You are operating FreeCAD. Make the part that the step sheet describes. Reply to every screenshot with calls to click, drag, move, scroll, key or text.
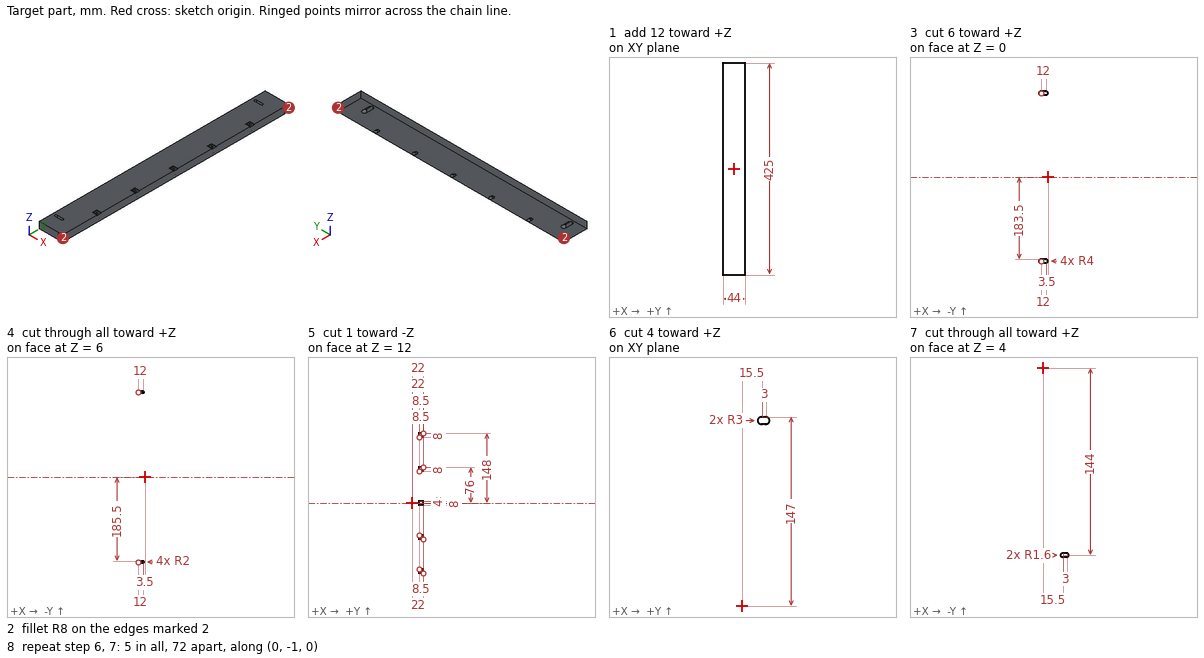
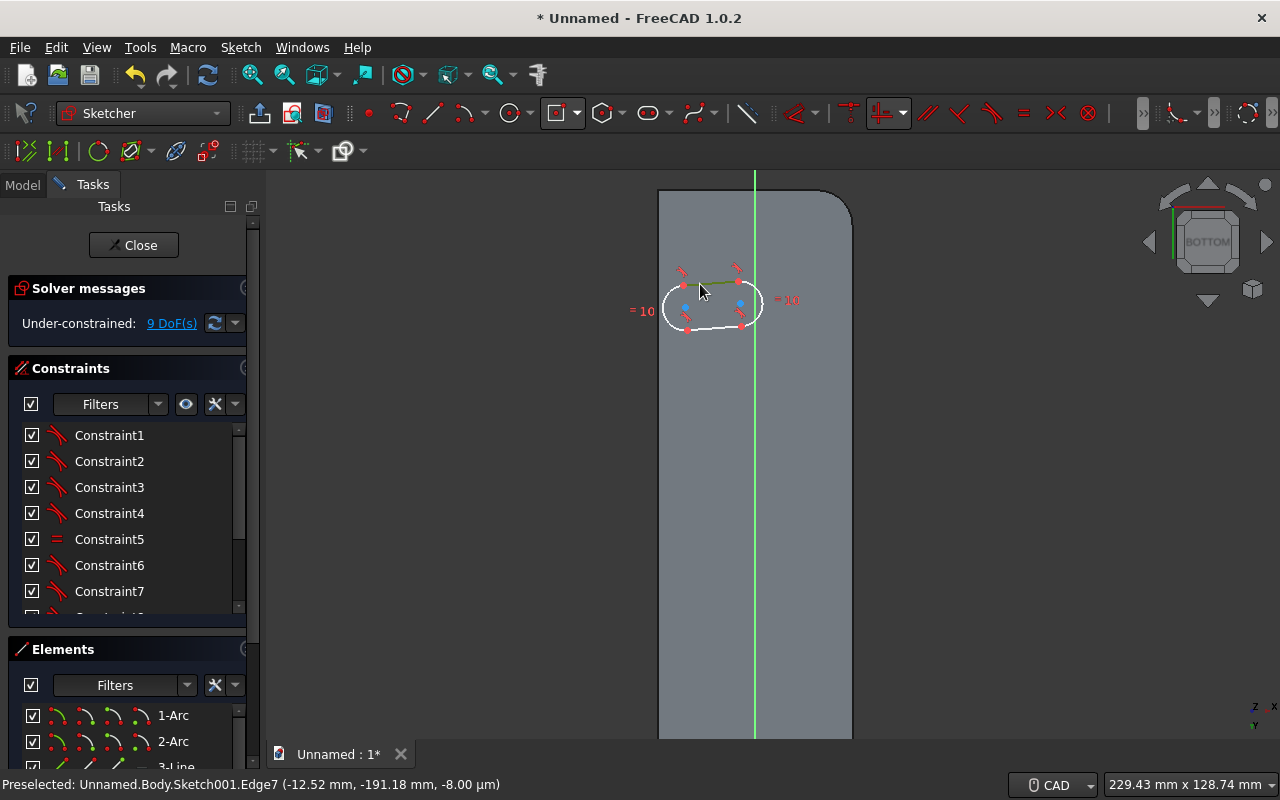
key(h)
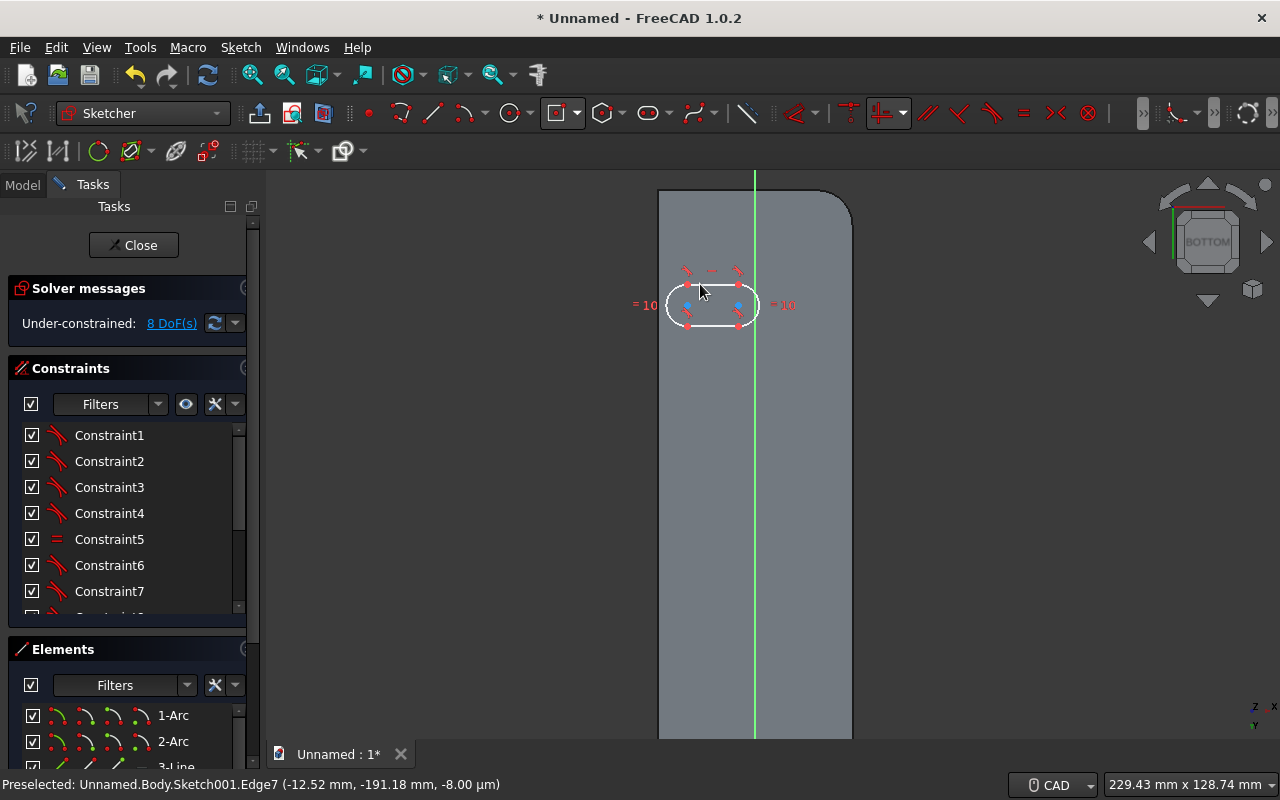
scroll(702, 284, down, 8)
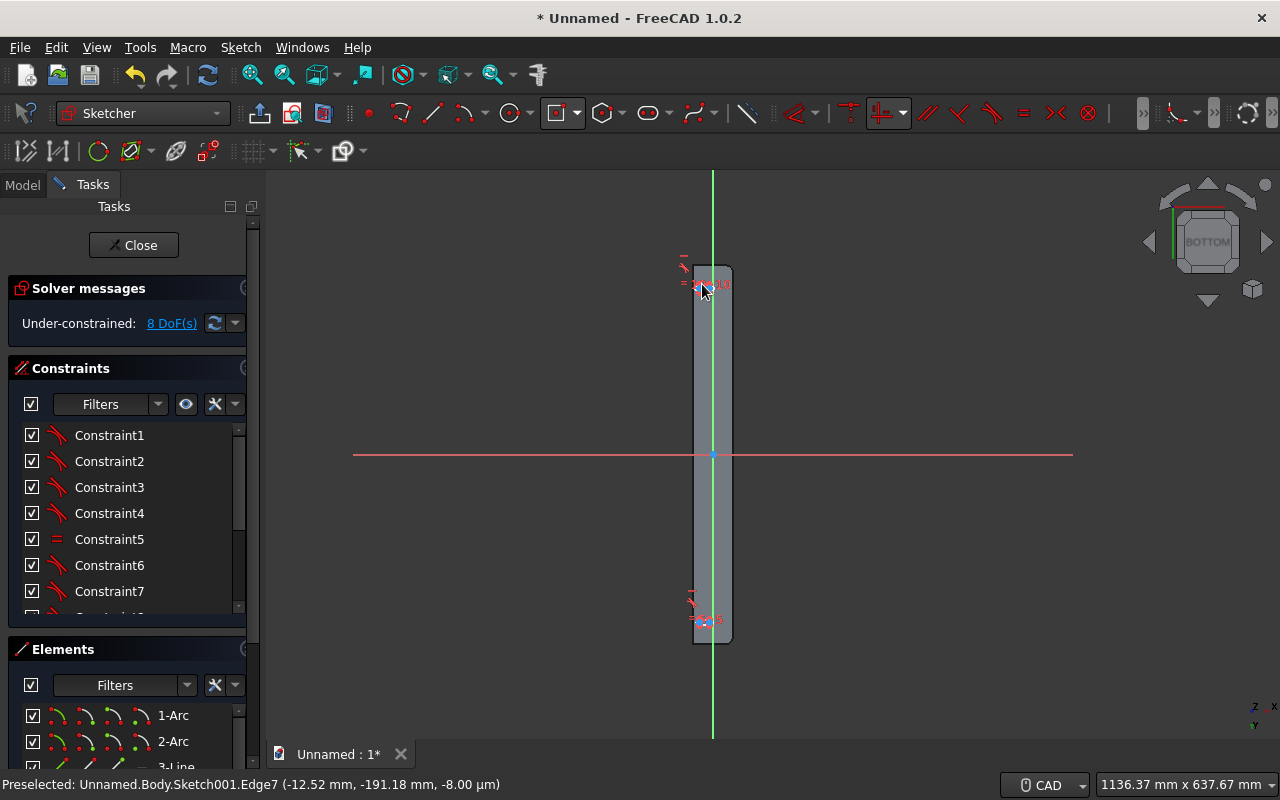
scroll(697, 621, up, 9)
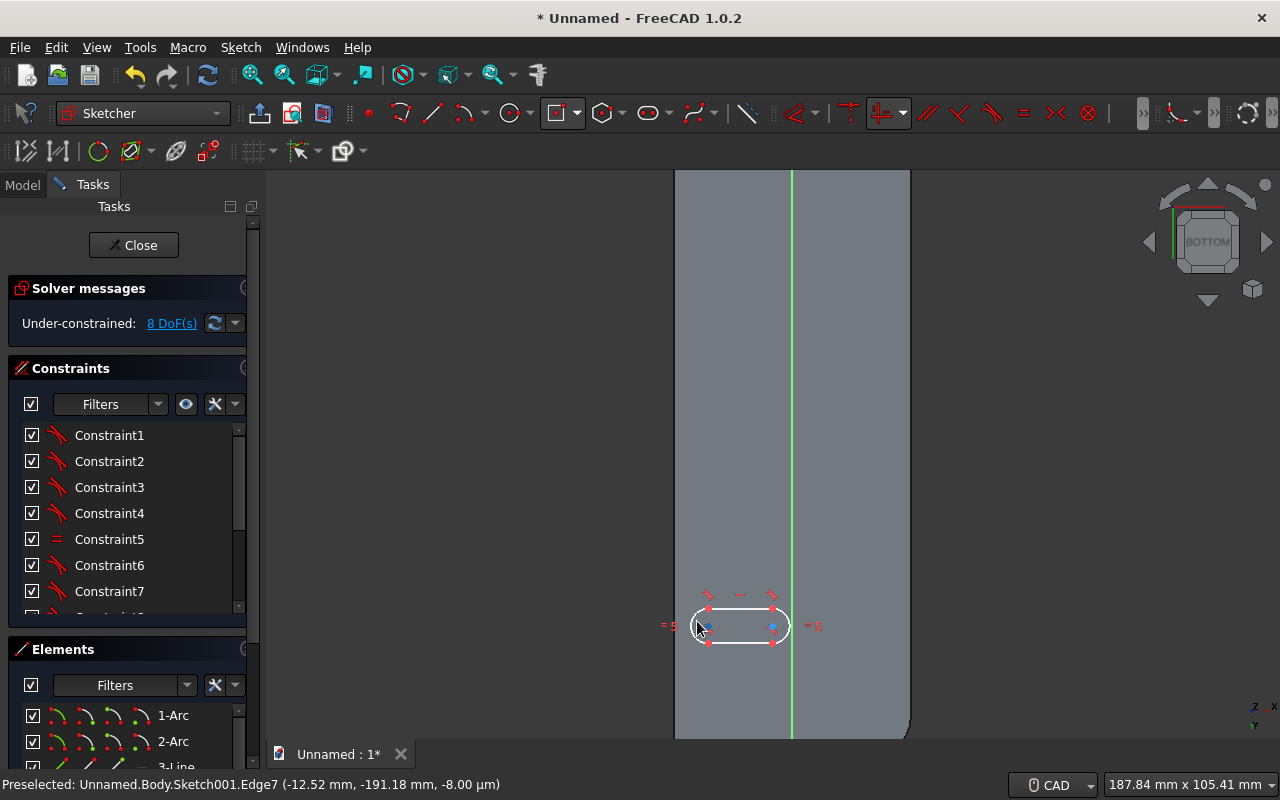
click(694, 616)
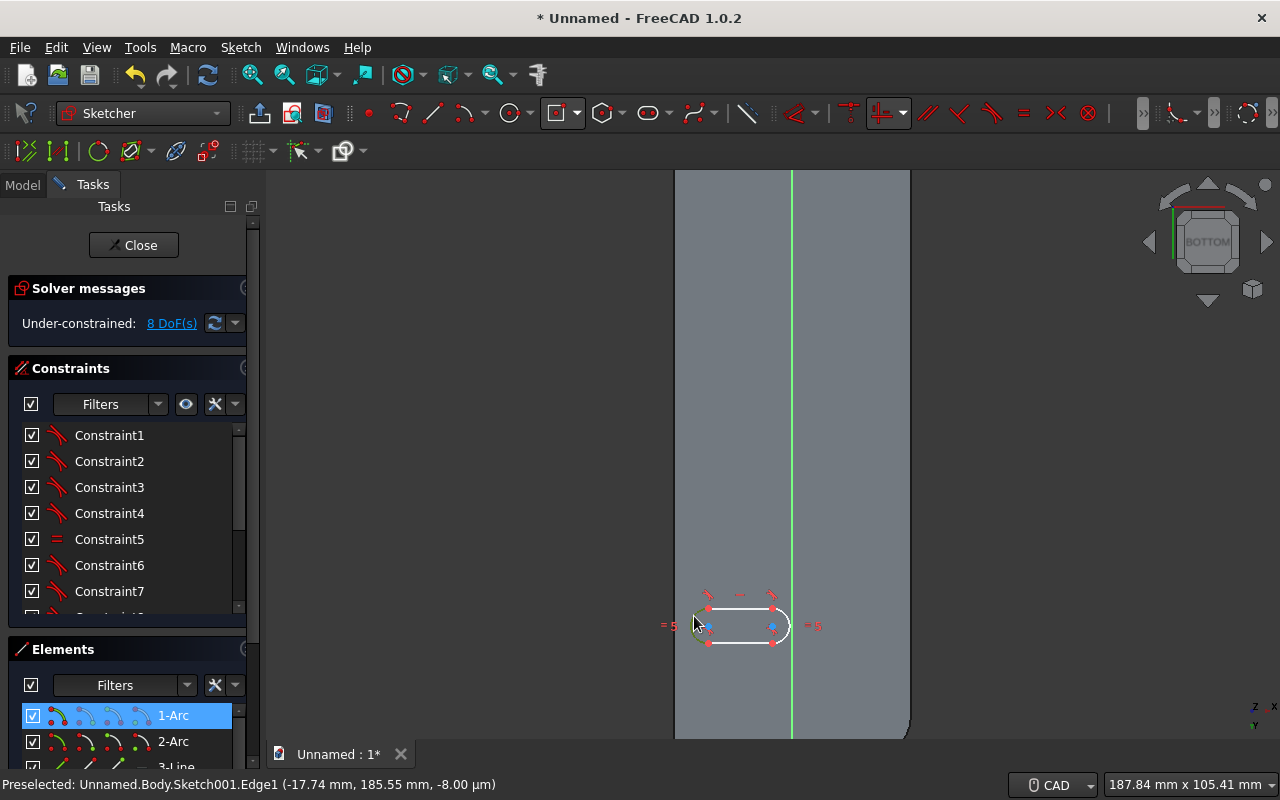
scroll(697, 621, down, 9)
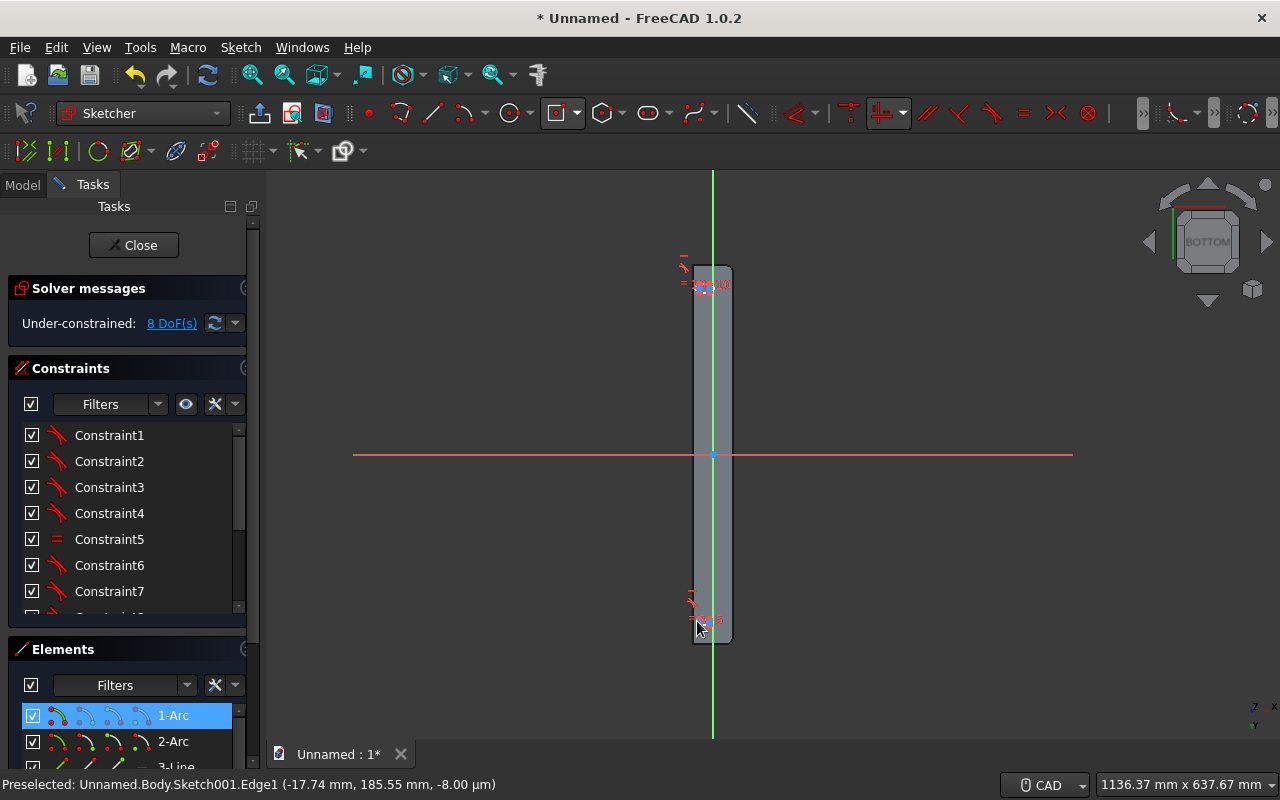
scroll(696, 286, up, 7)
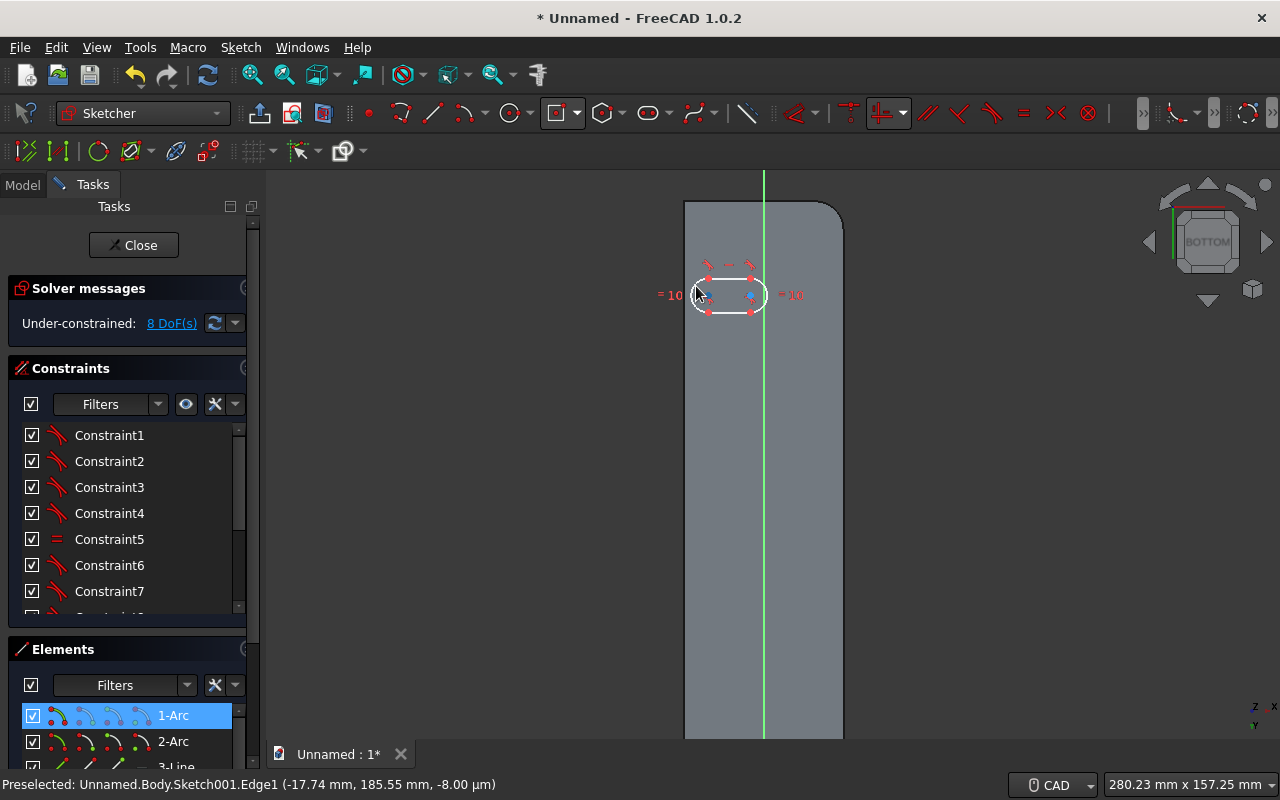
click(695, 286)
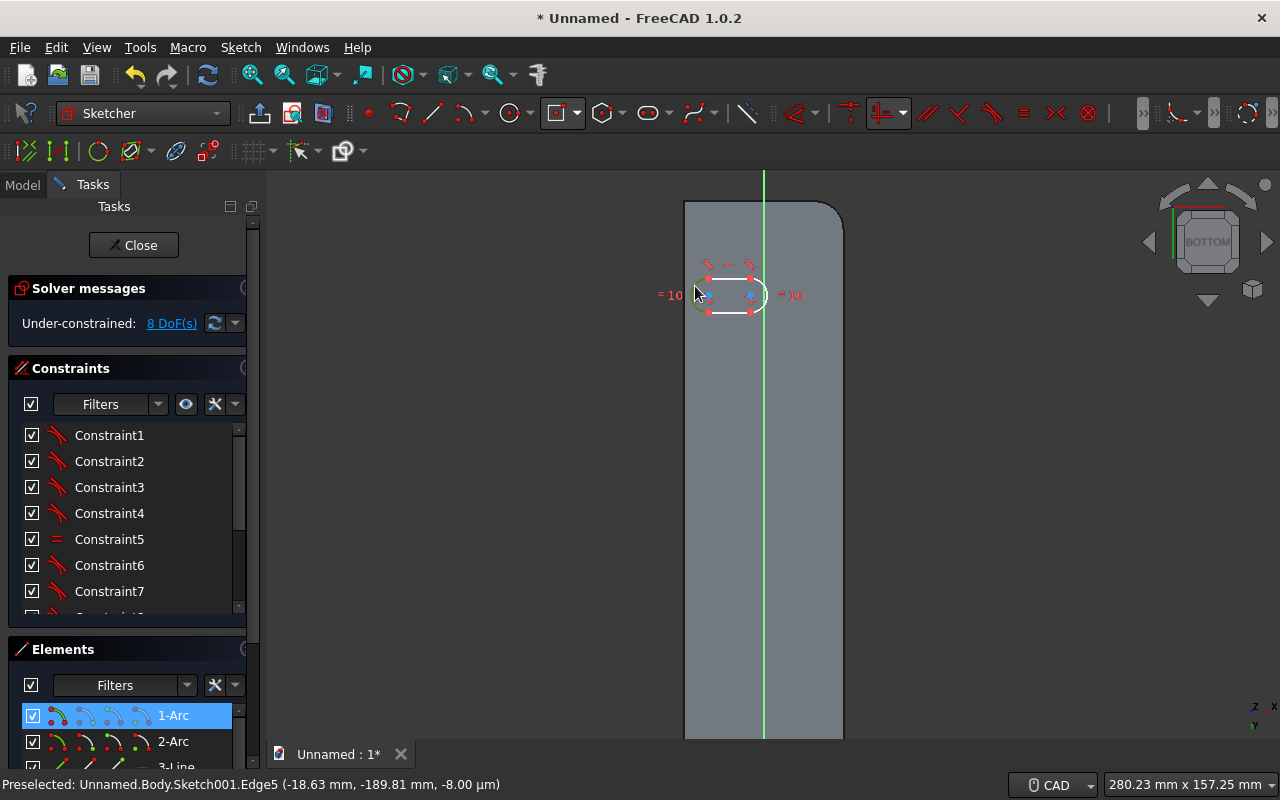
click(1024, 114)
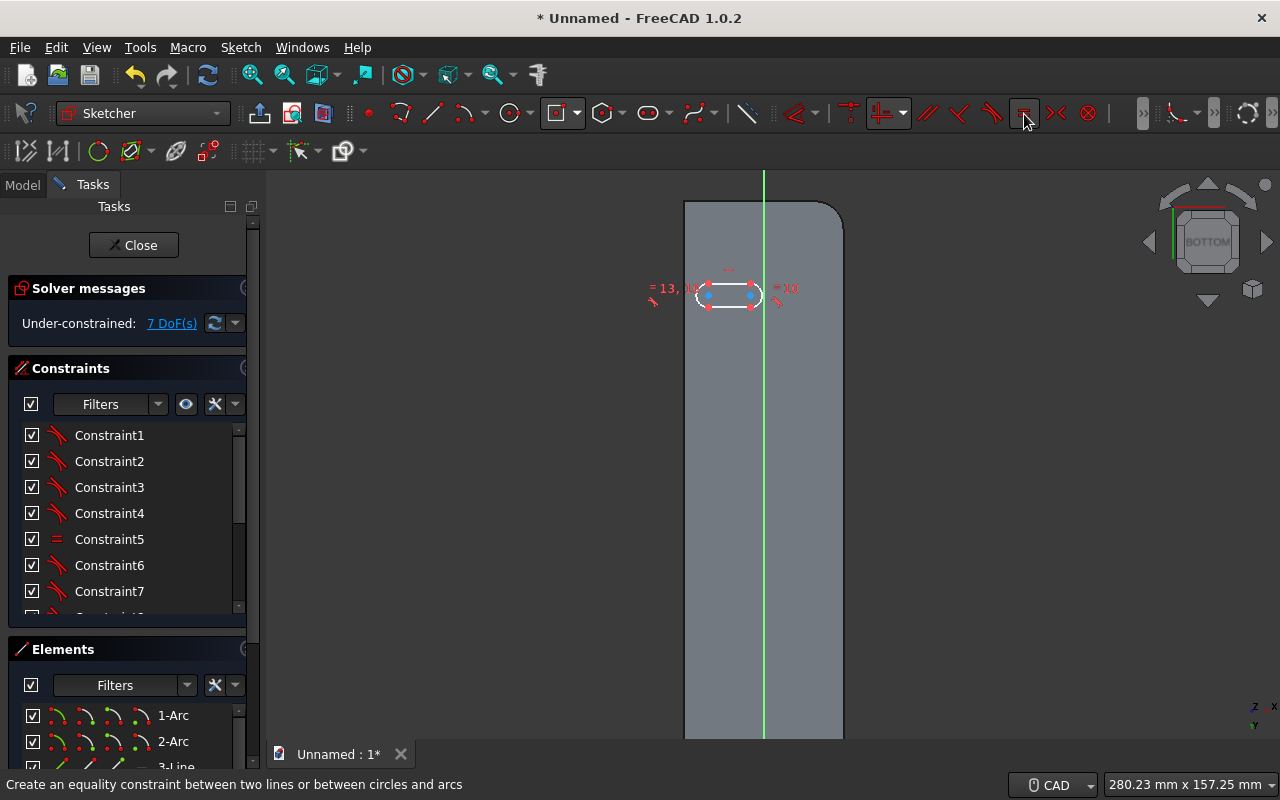
scroll(696, 286, down, 7)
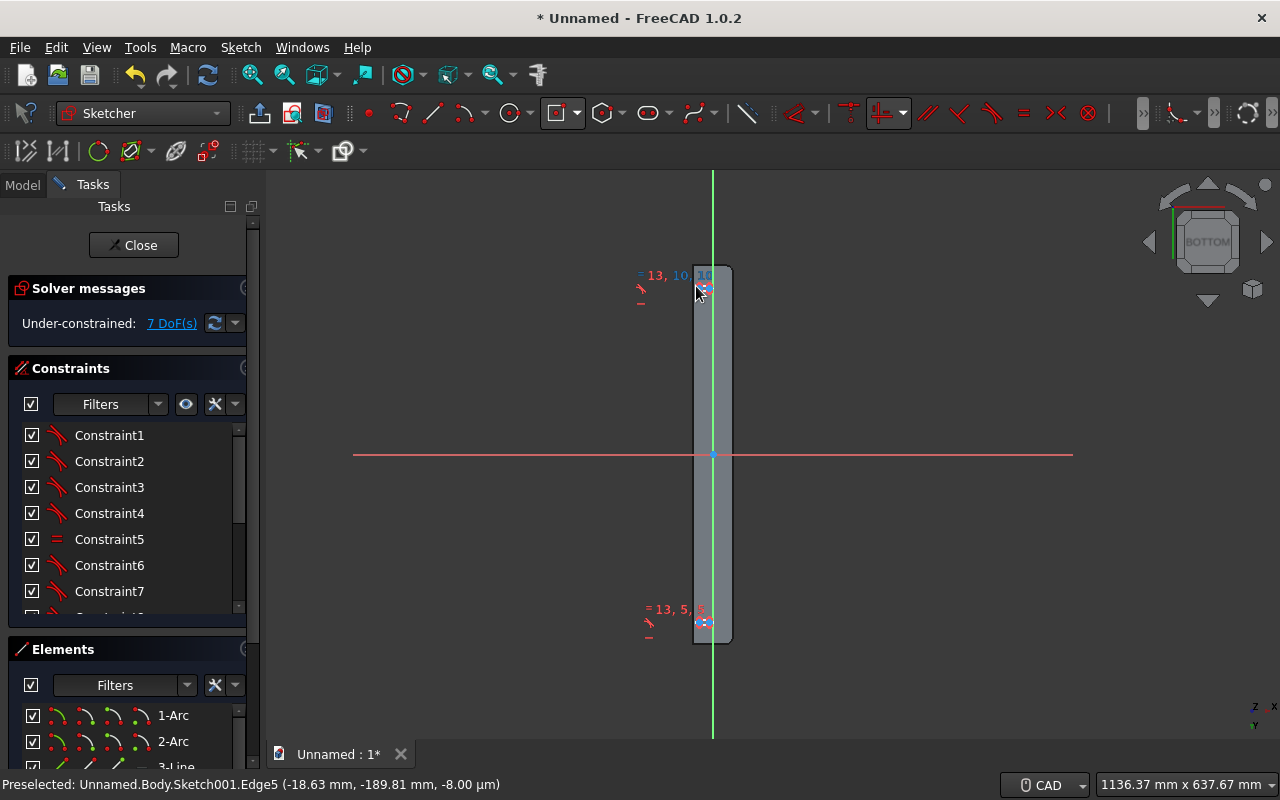
scroll(699, 622, up, 8)